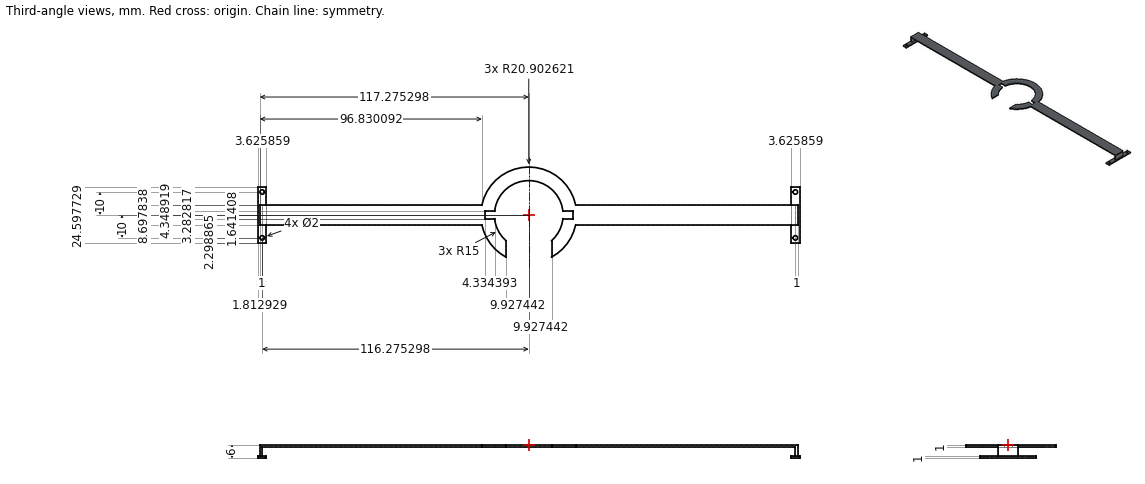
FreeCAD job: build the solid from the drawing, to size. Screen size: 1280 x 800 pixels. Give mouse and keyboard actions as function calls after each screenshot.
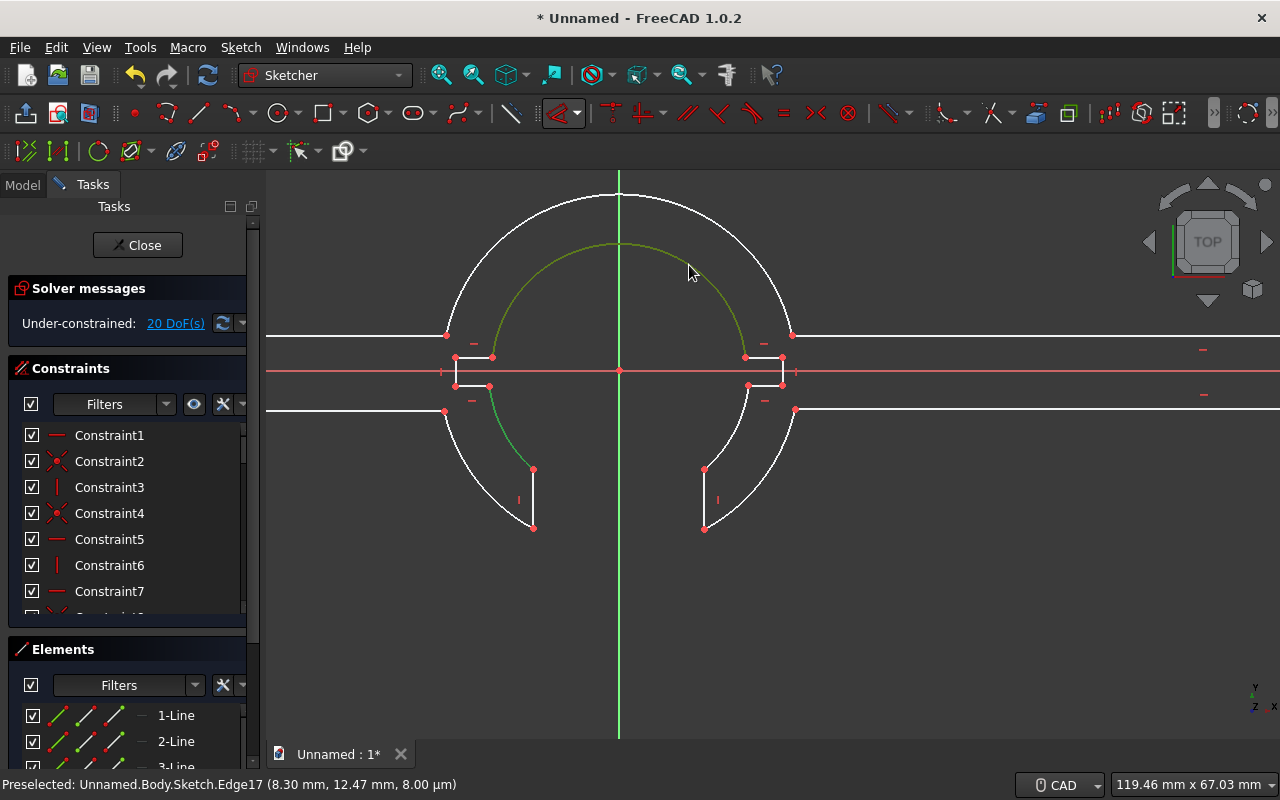
click(724, 449)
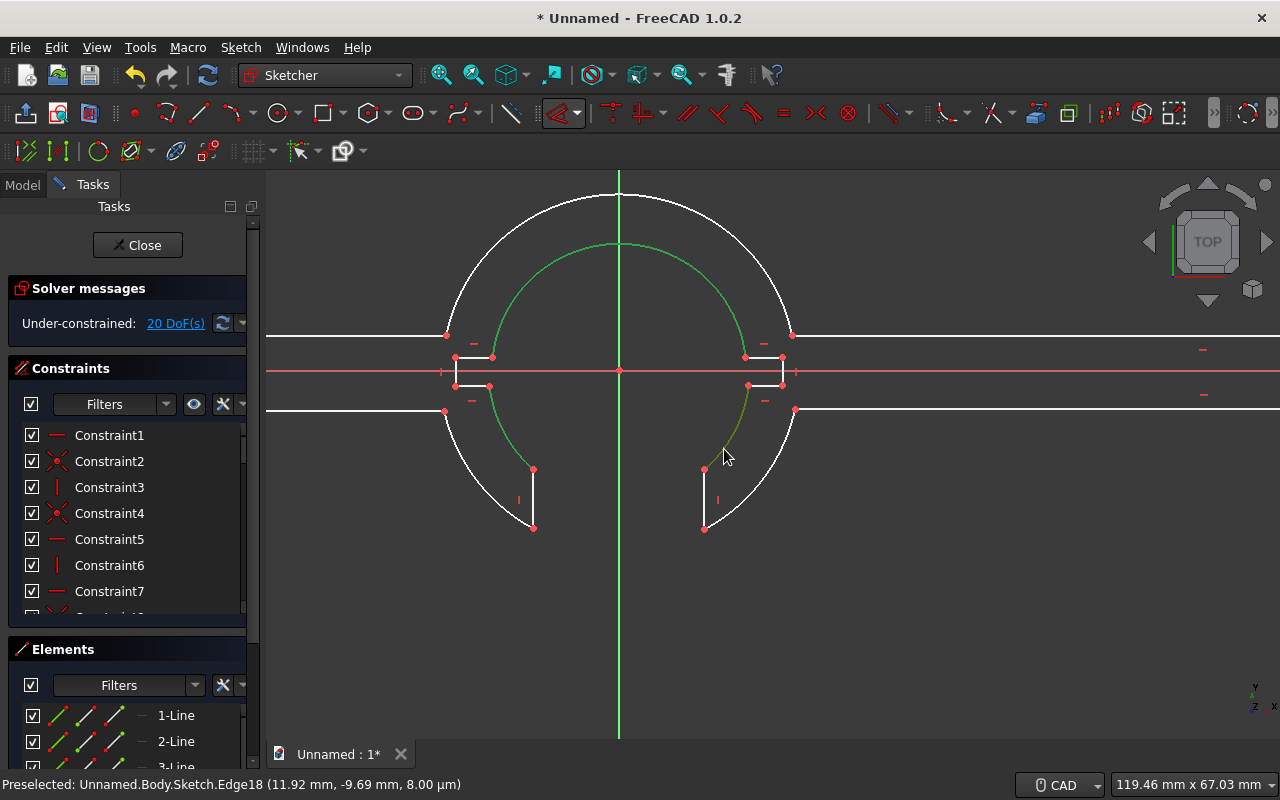
click(784, 114)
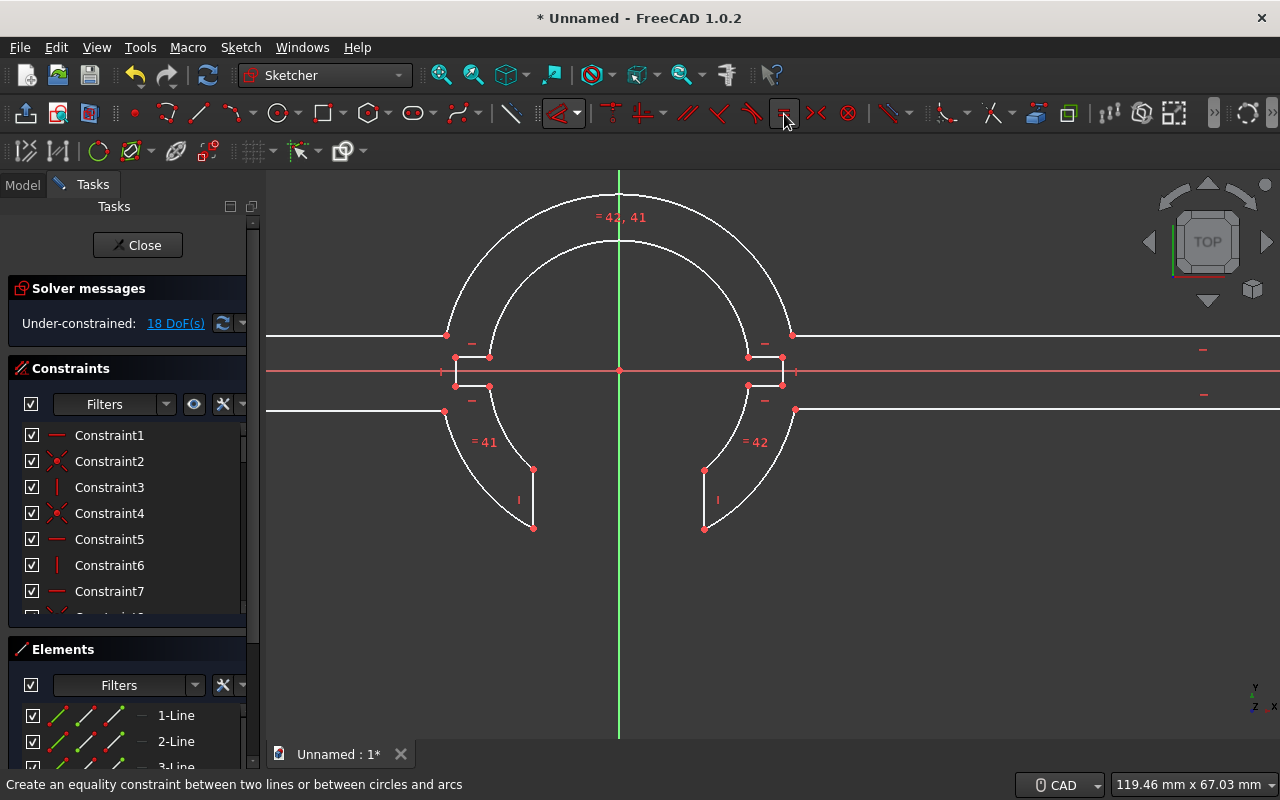
click(460, 454)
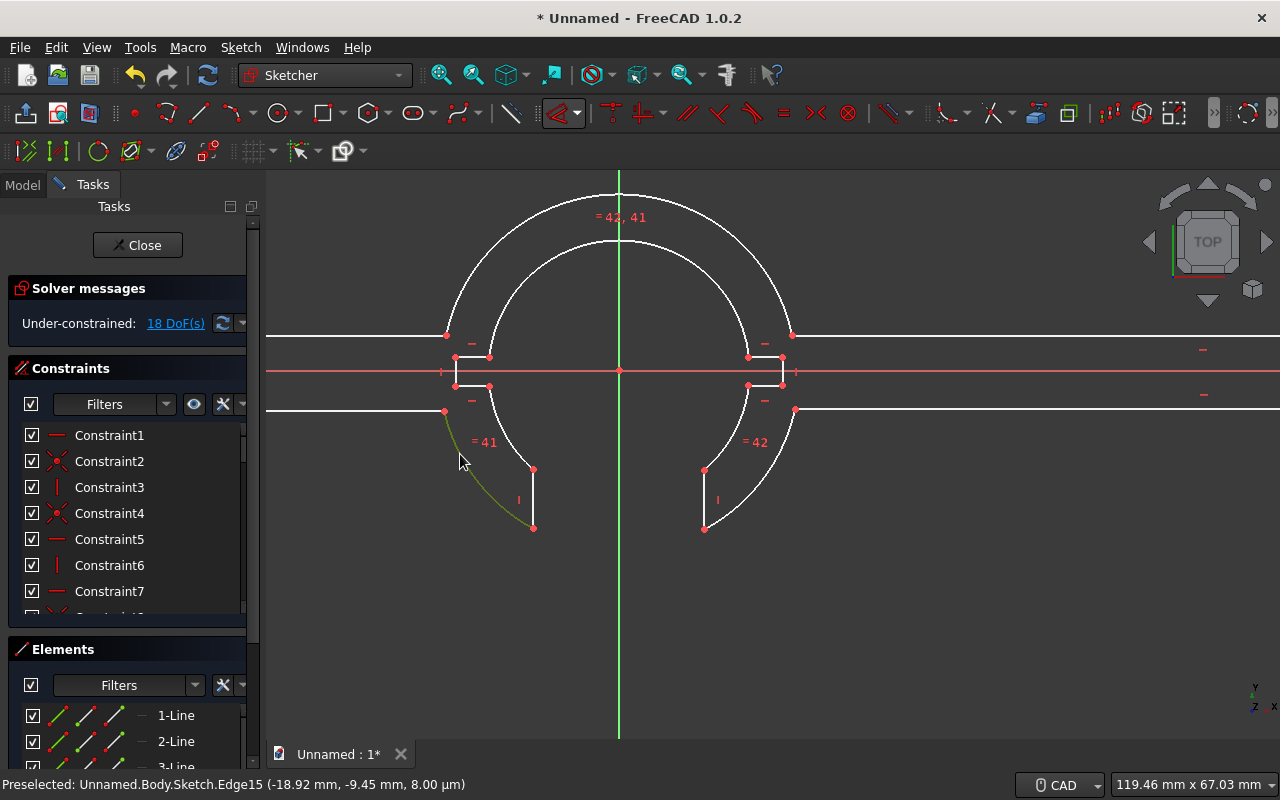
click(742, 503)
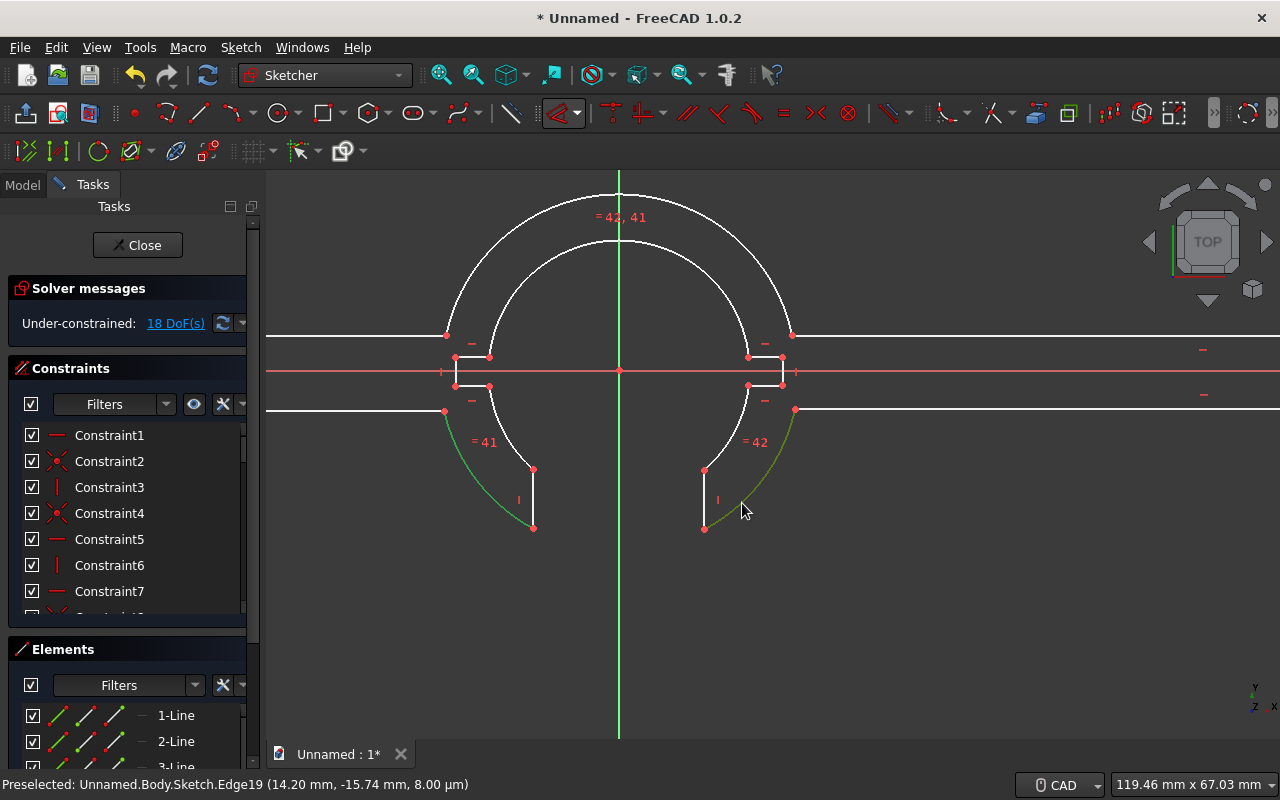
click(711, 220)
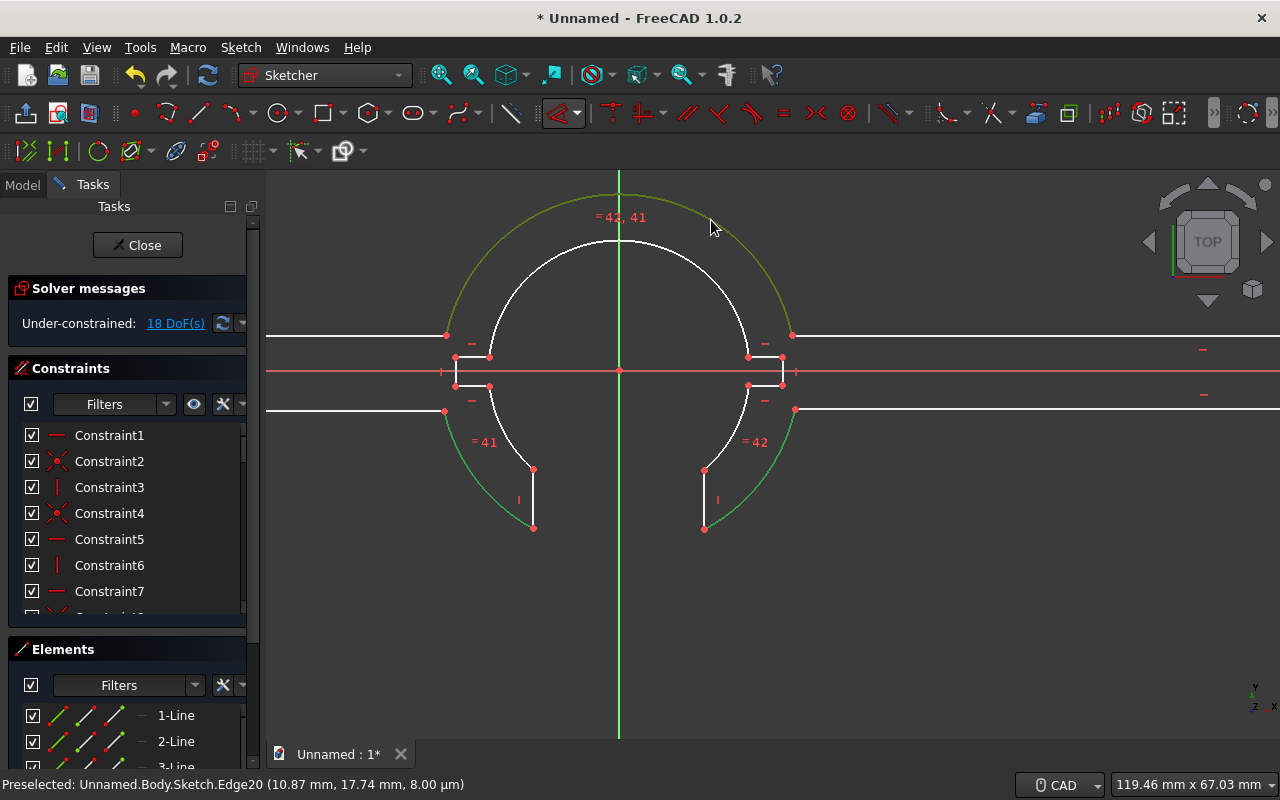
click(784, 114)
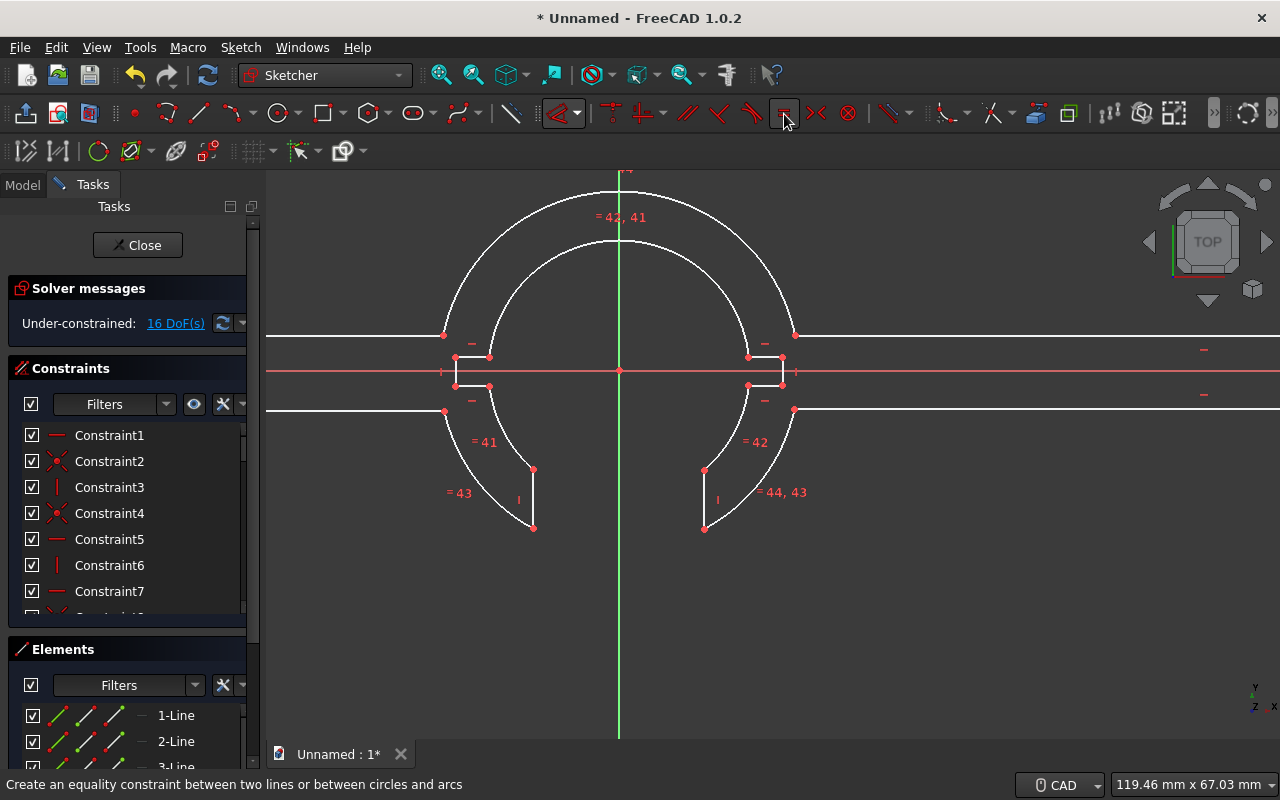
click(456, 357)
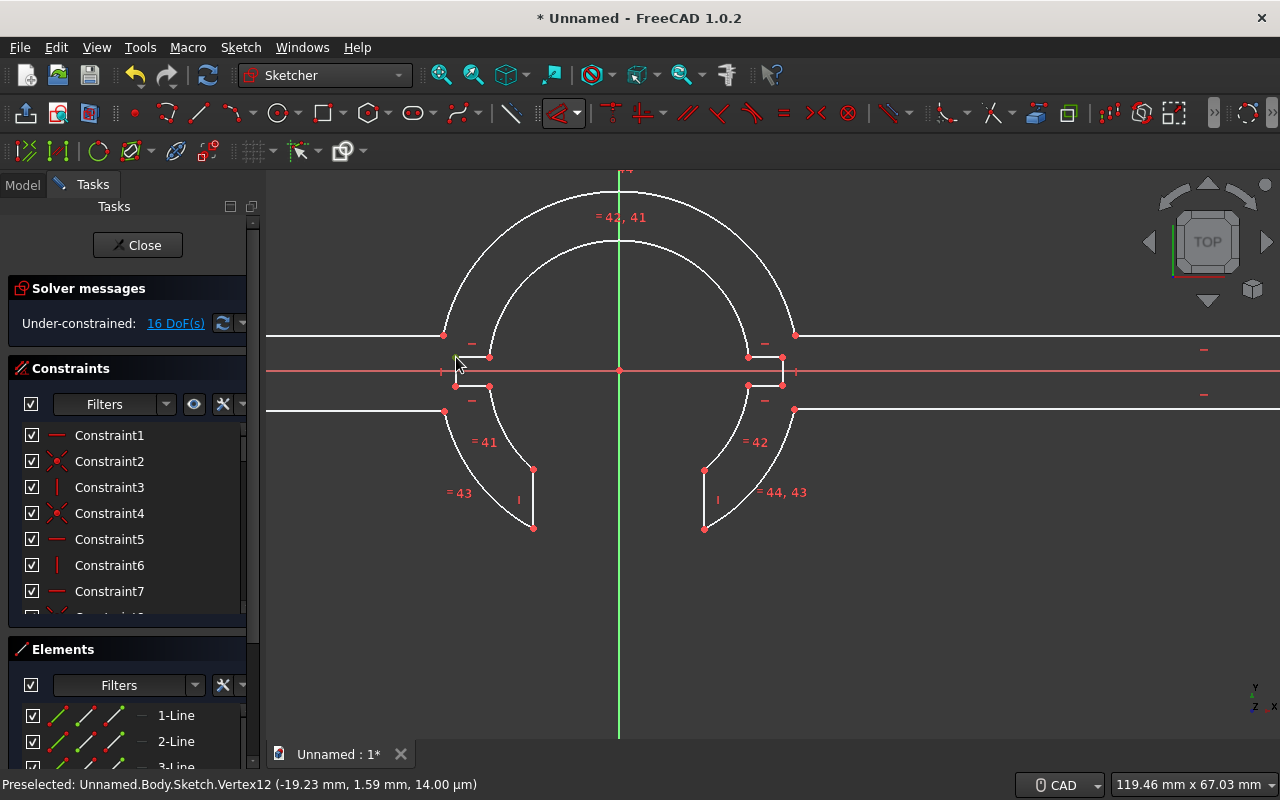
click(783, 357)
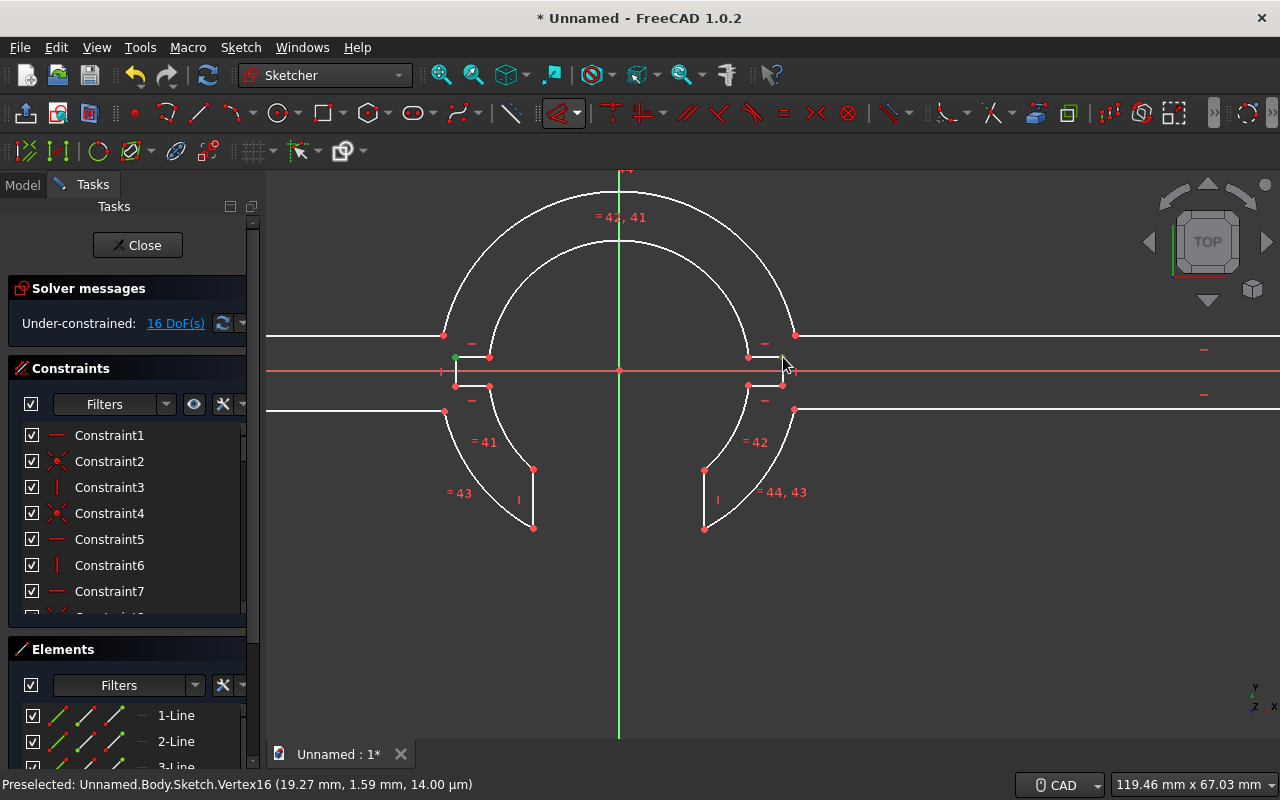
click(619, 674)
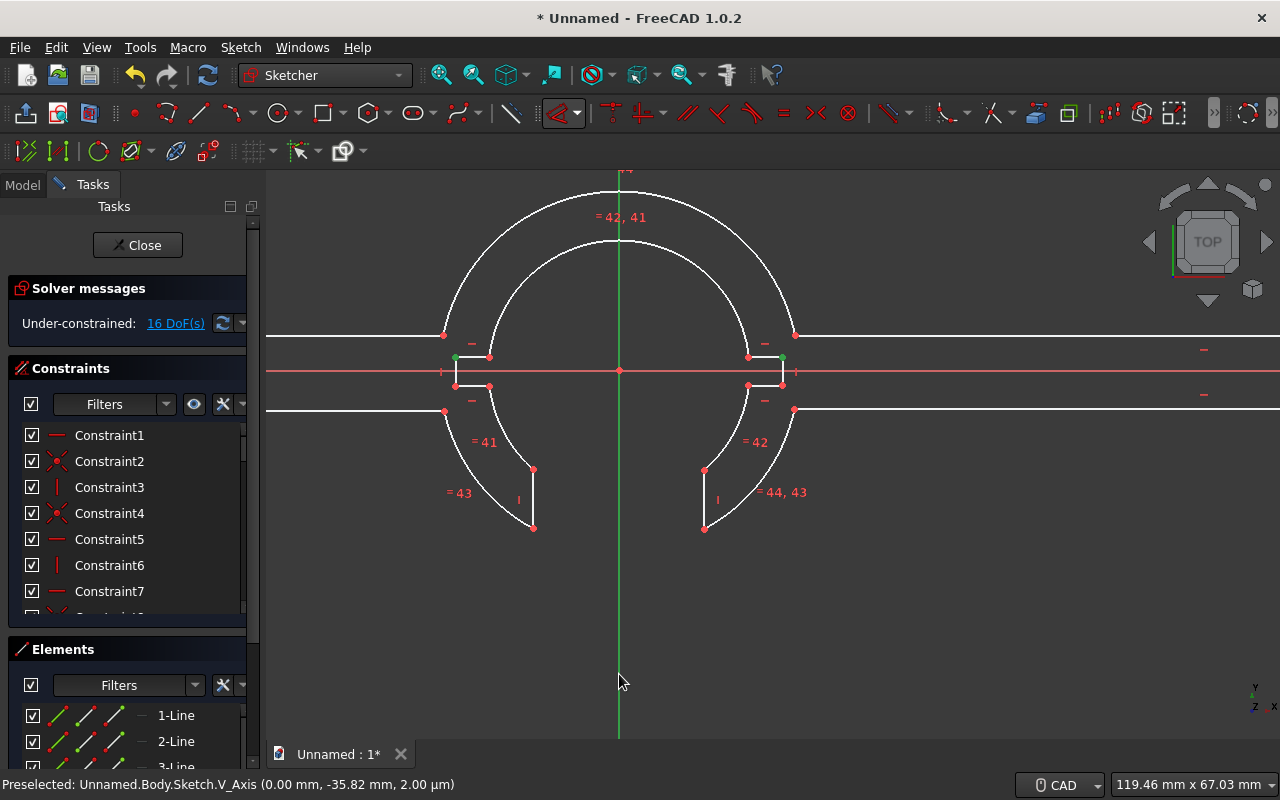
key(s)